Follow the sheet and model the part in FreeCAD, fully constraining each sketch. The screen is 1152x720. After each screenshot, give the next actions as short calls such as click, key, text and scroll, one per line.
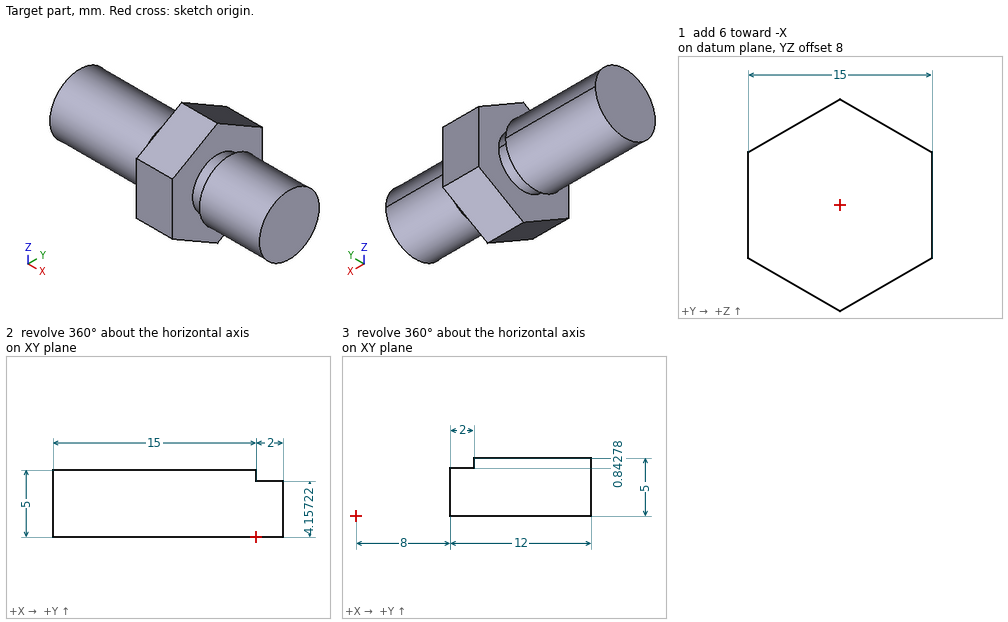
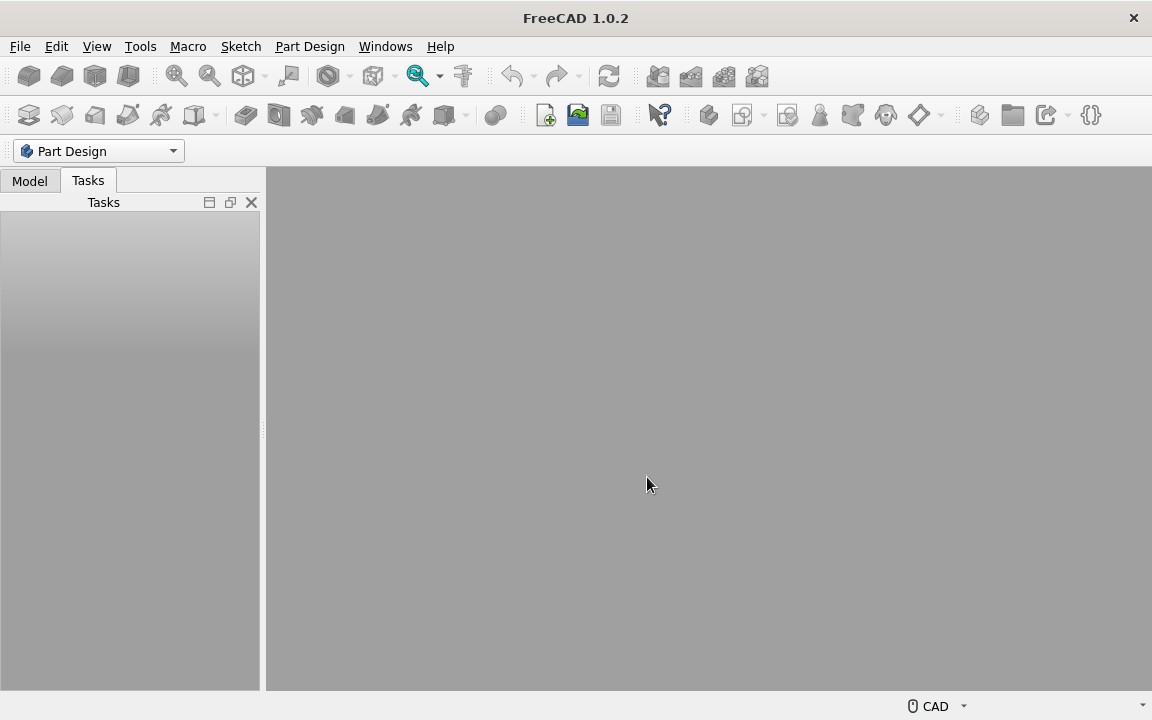
click(545, 116)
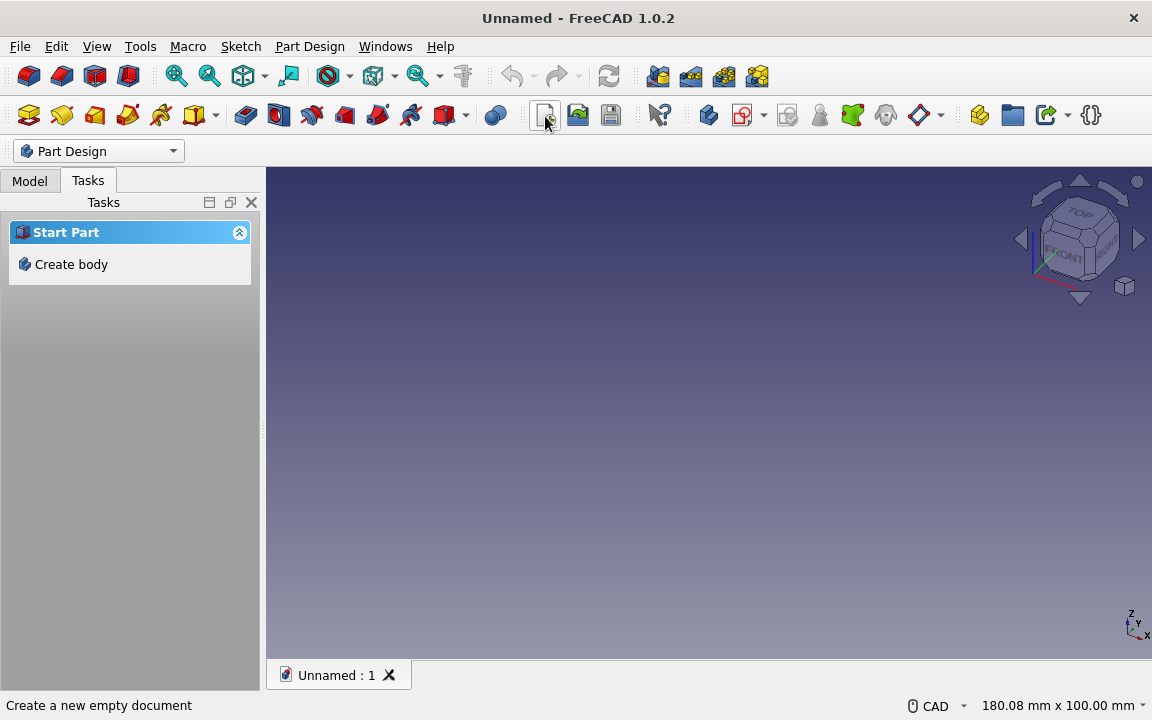
click(709, 116)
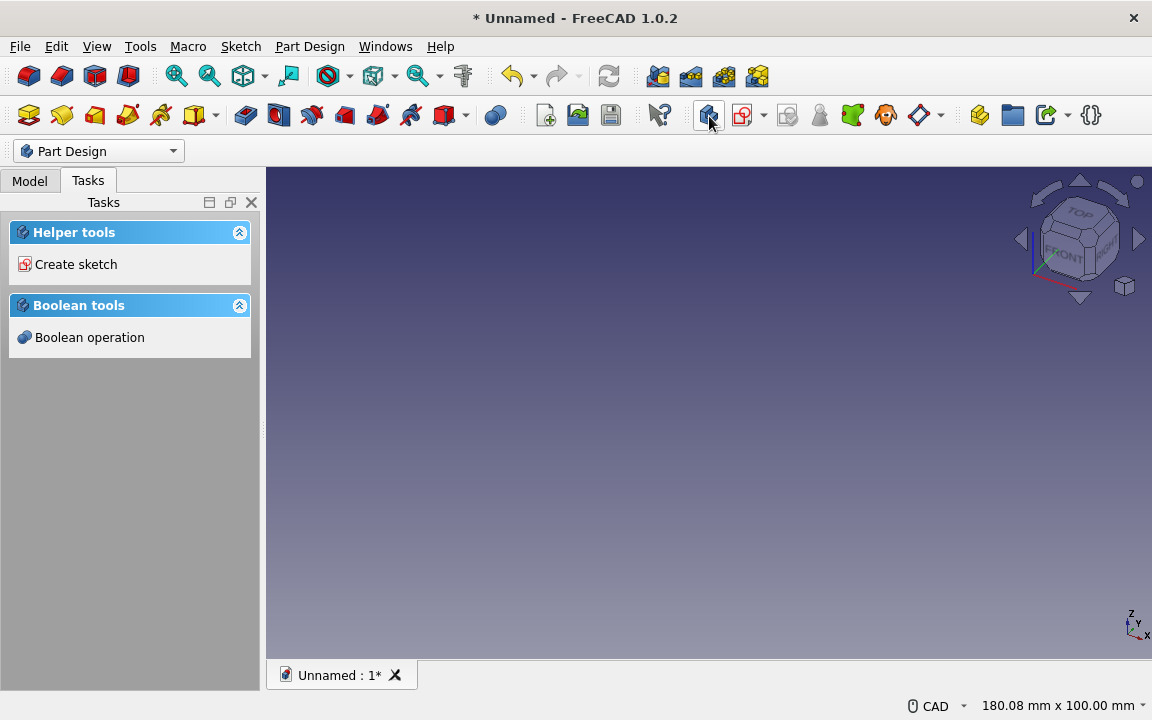
click(30, 180)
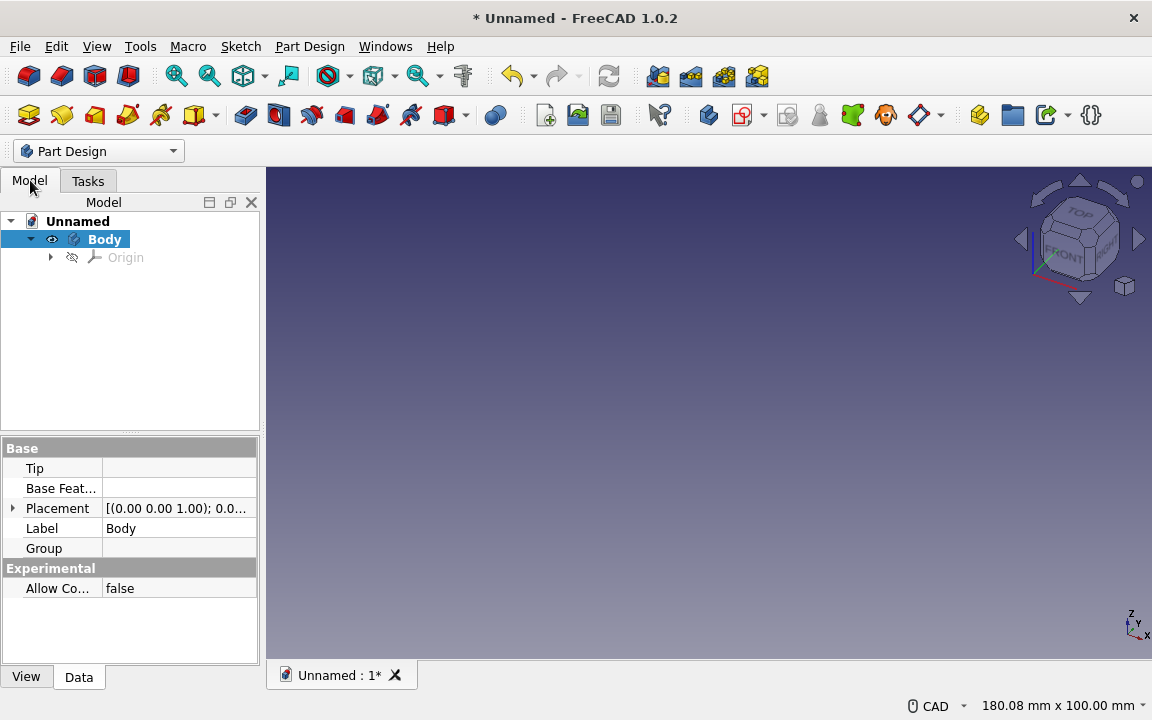
click(51, 257)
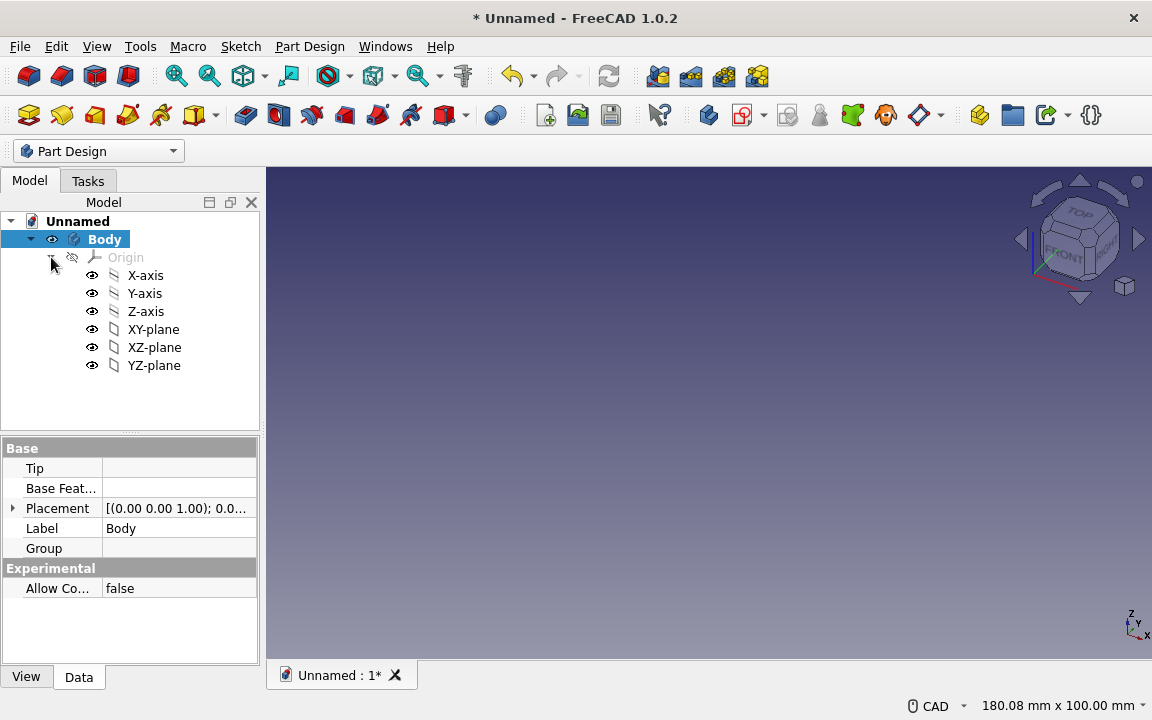
click(137, 365)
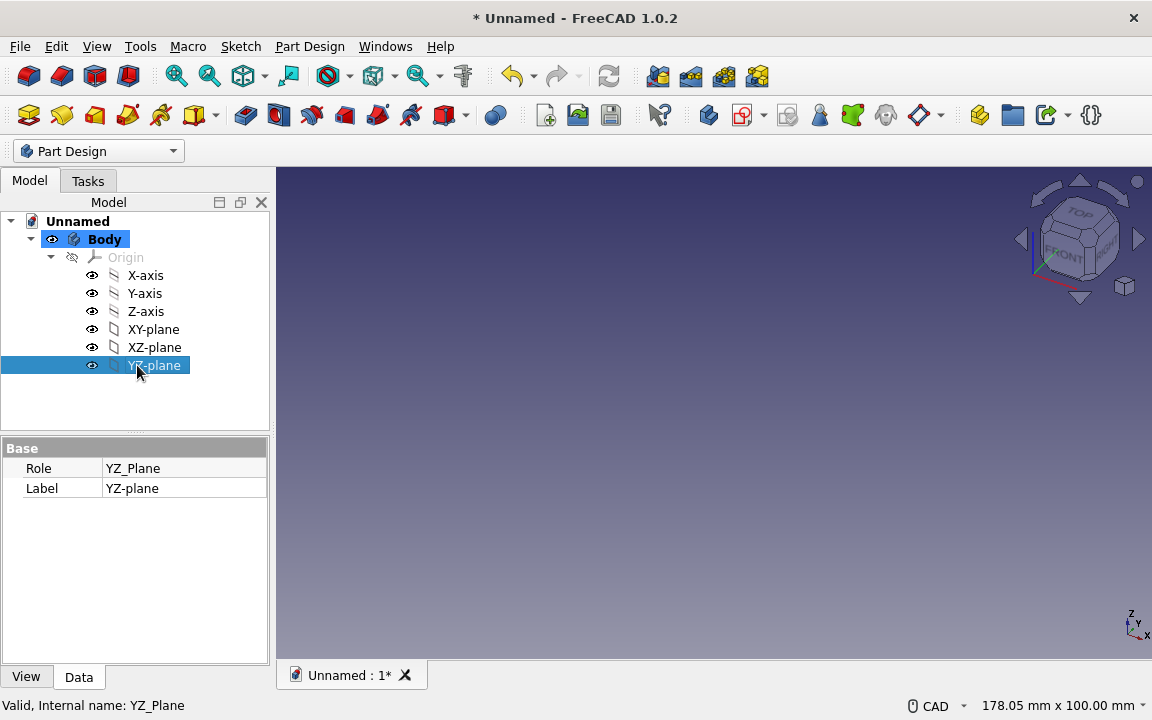
click(918, 116)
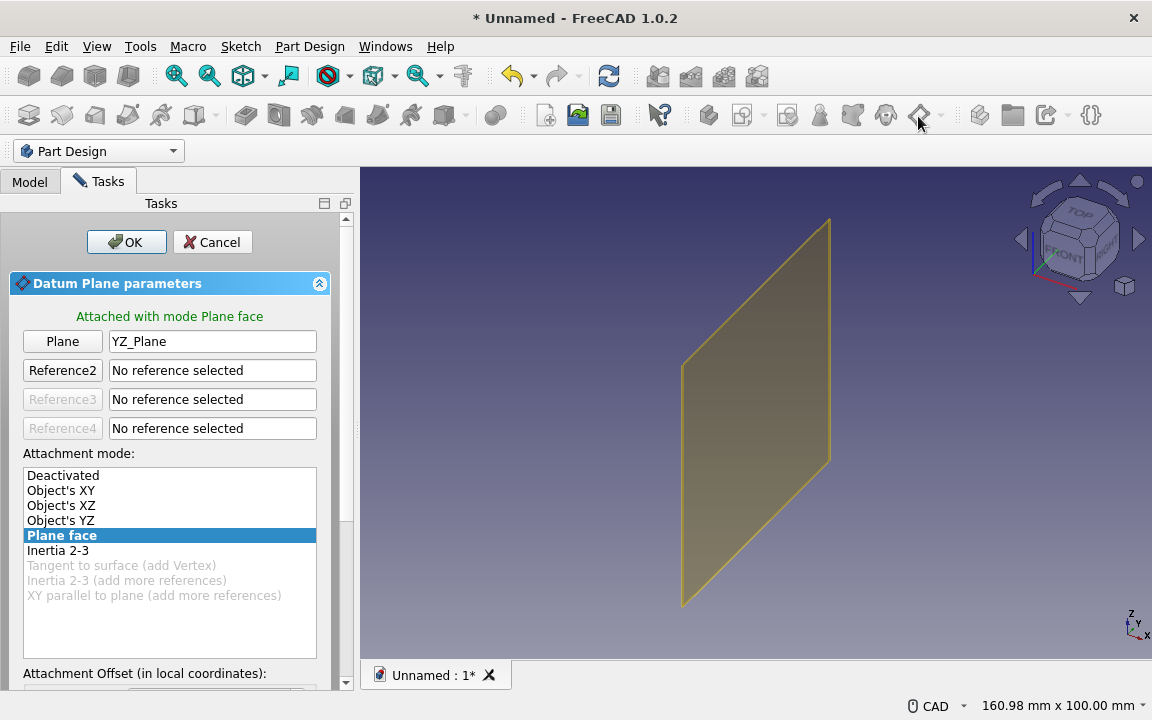
scroll(346, 452, down, 3)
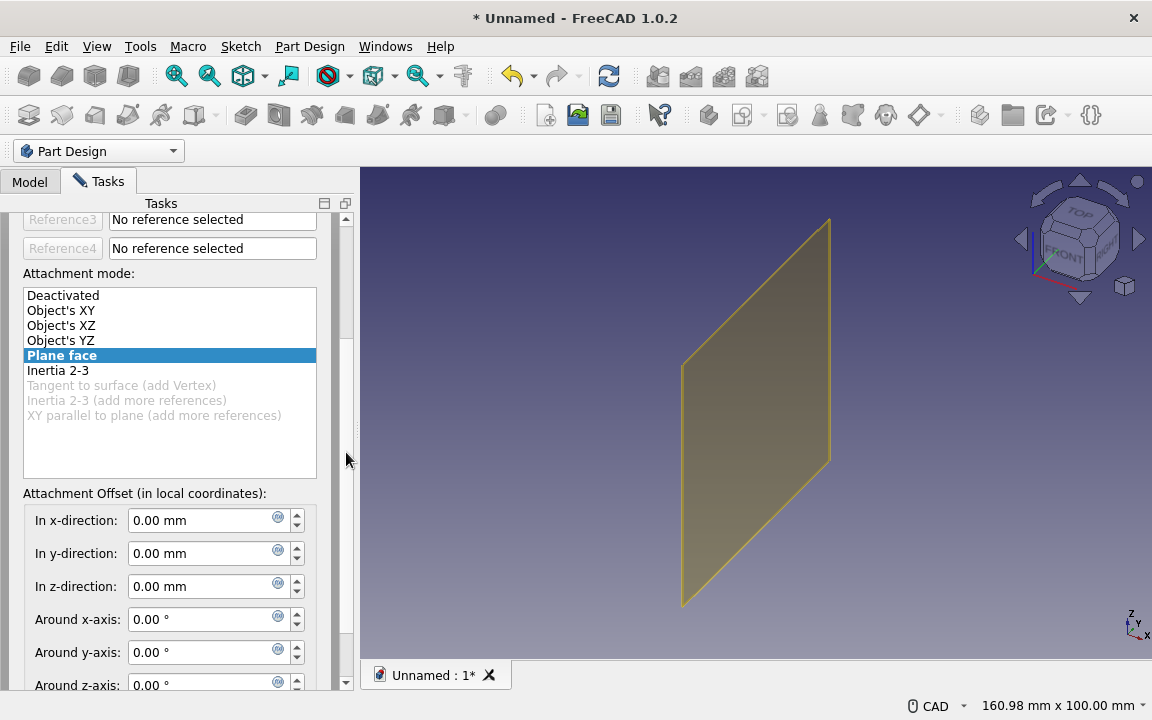
triple_click(210, 586)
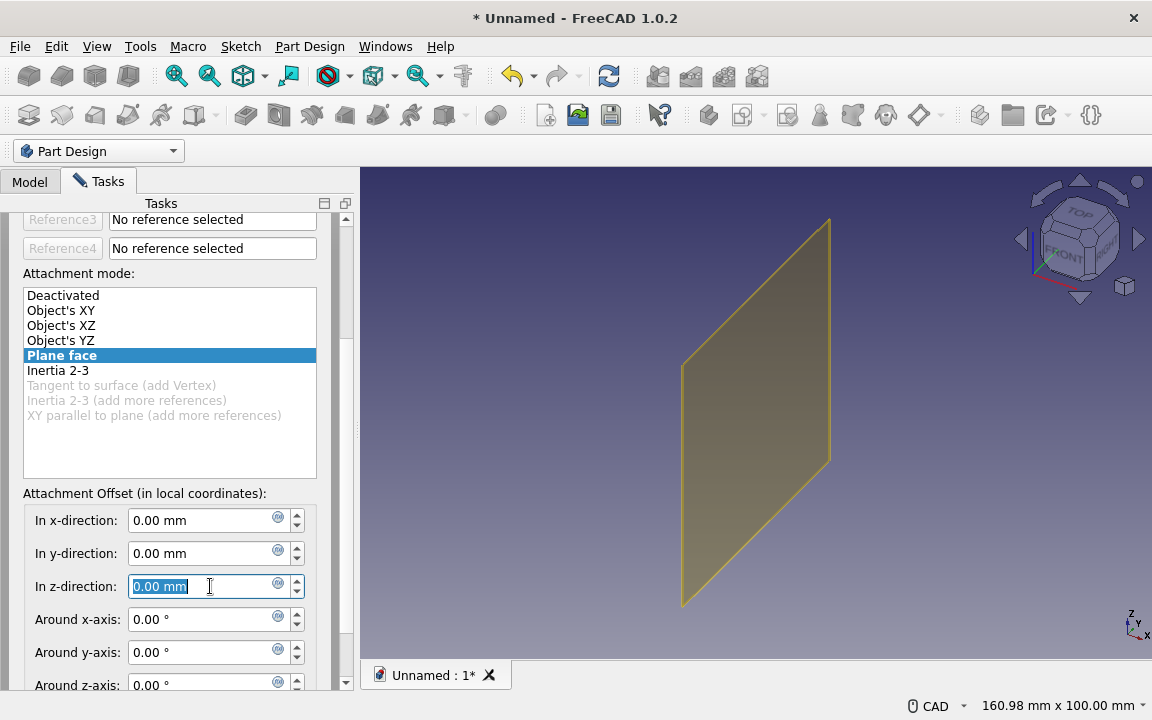
text(8)
key(Tab)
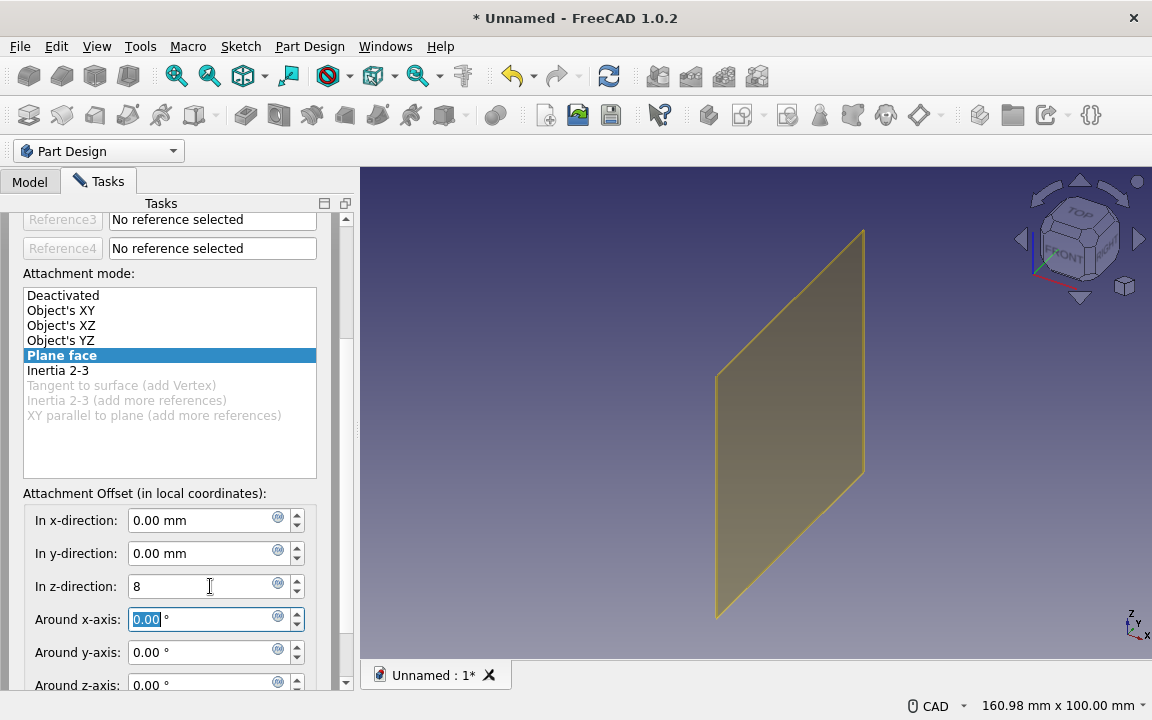
scroll(346, 452, up, 4)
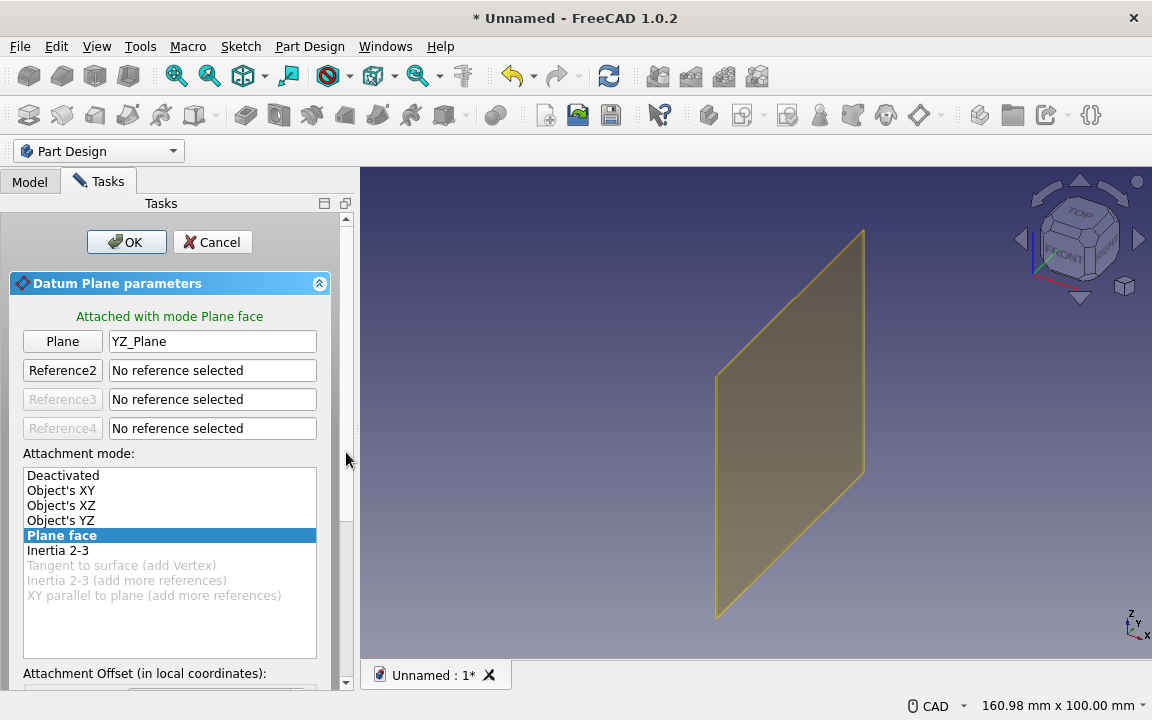
click(127, 242)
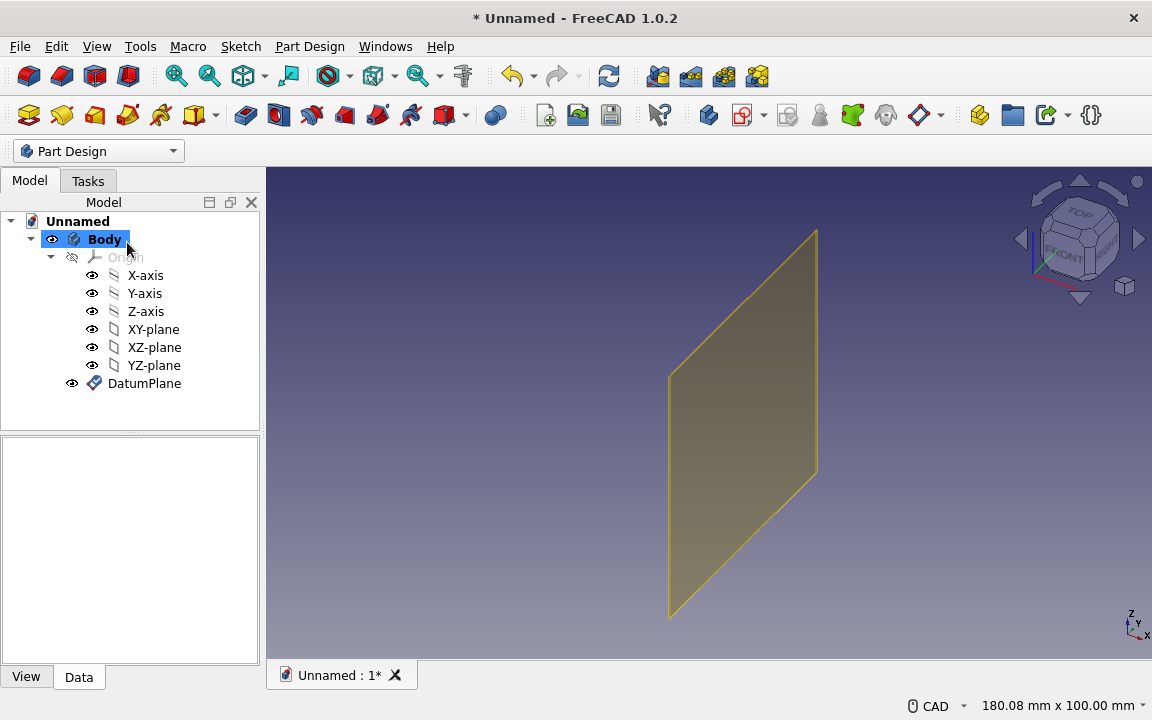
click(117, 383)